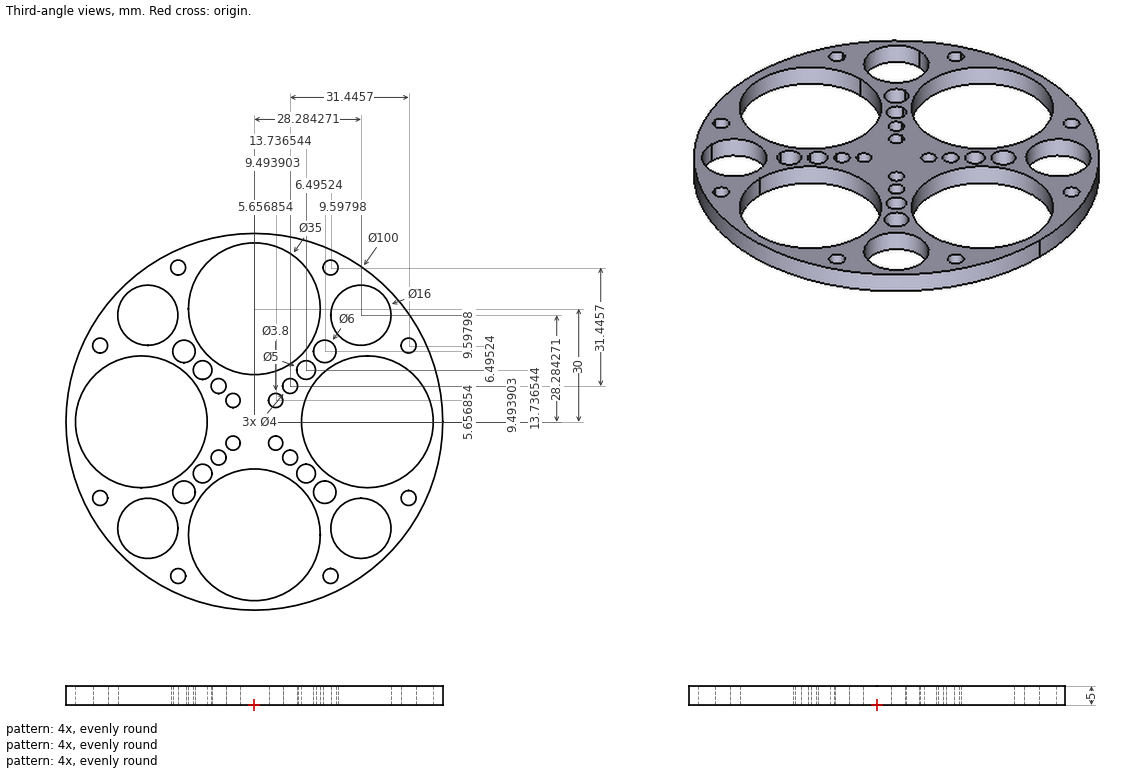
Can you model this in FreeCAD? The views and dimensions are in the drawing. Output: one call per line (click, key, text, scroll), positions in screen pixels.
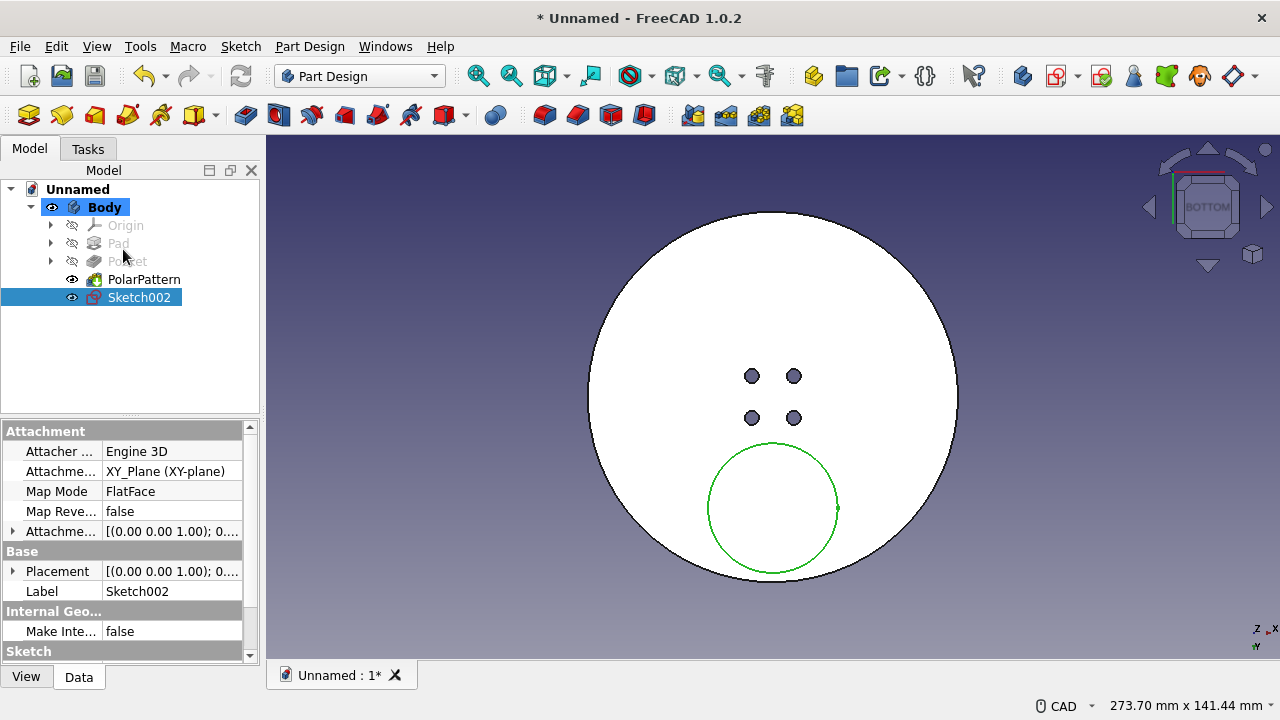
click(246, 116)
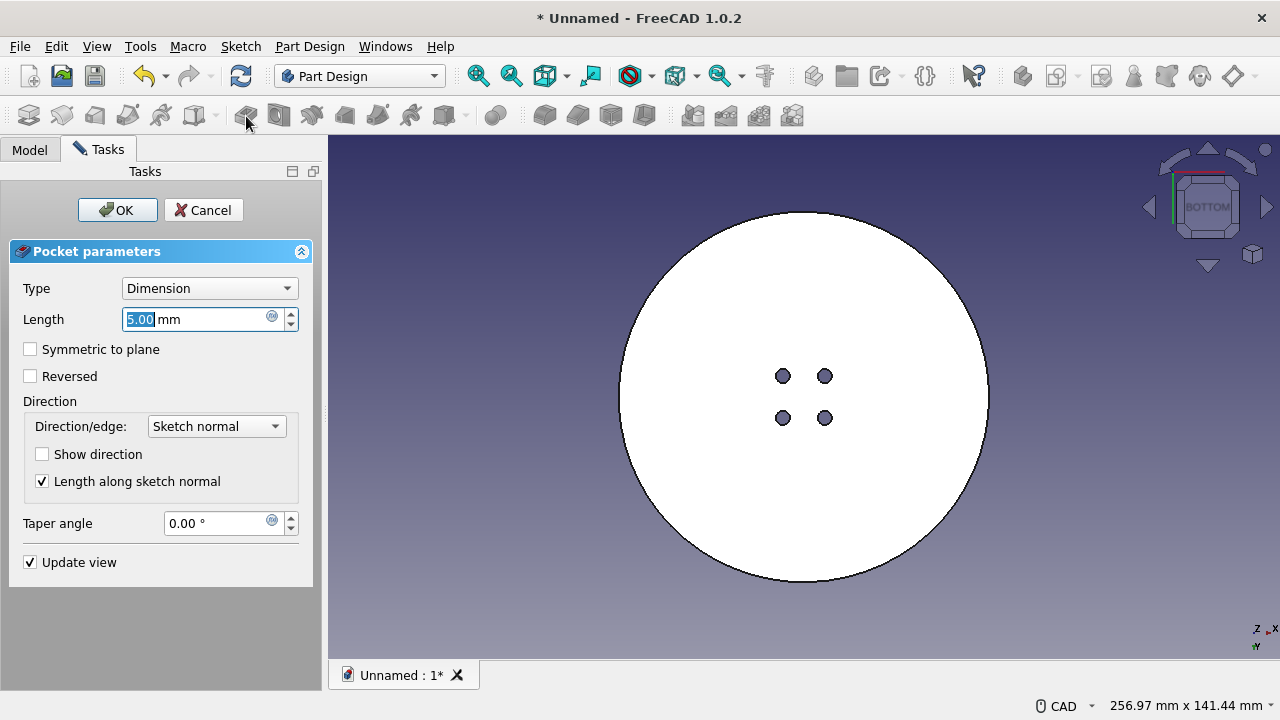
click(210, 288)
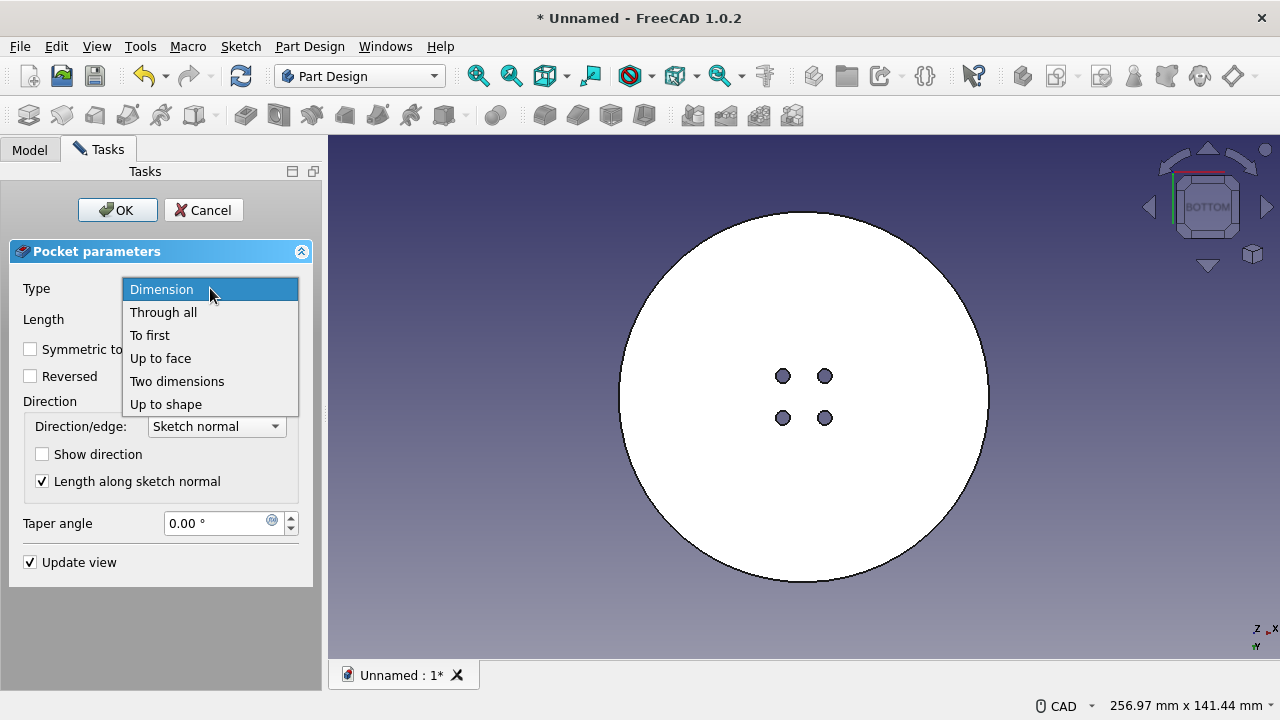
click(208, 312)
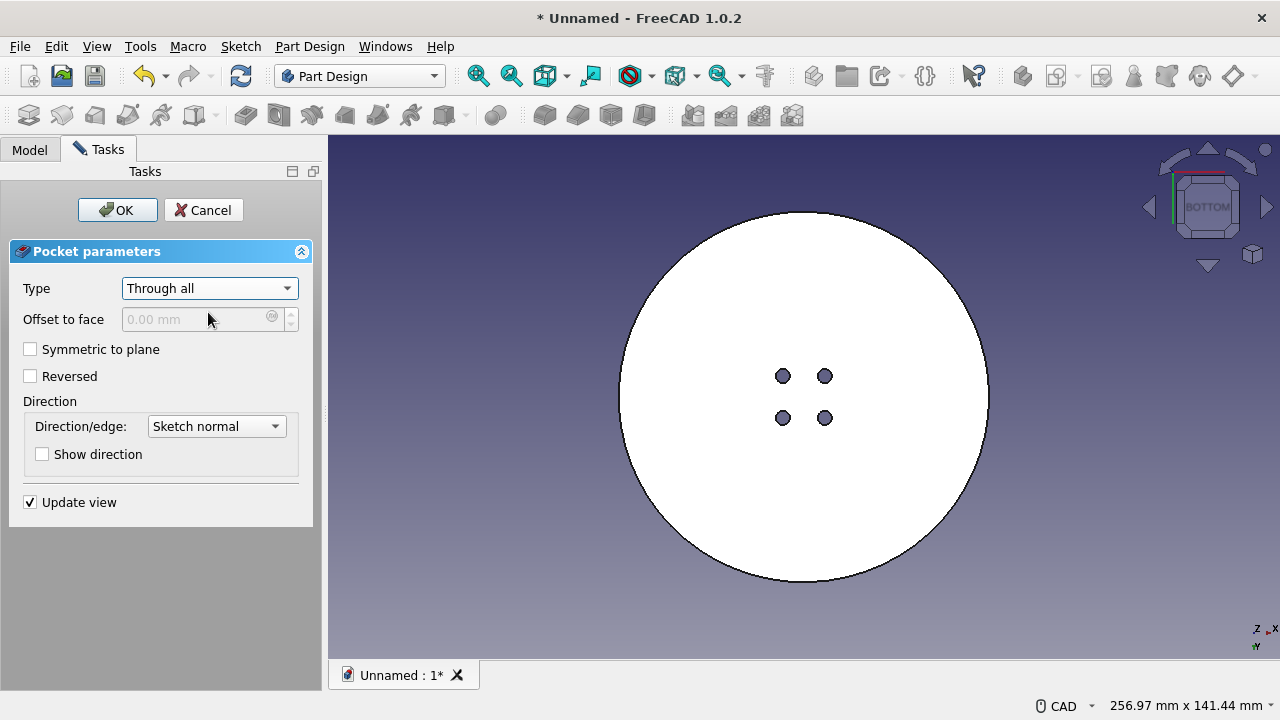
click(31, 376)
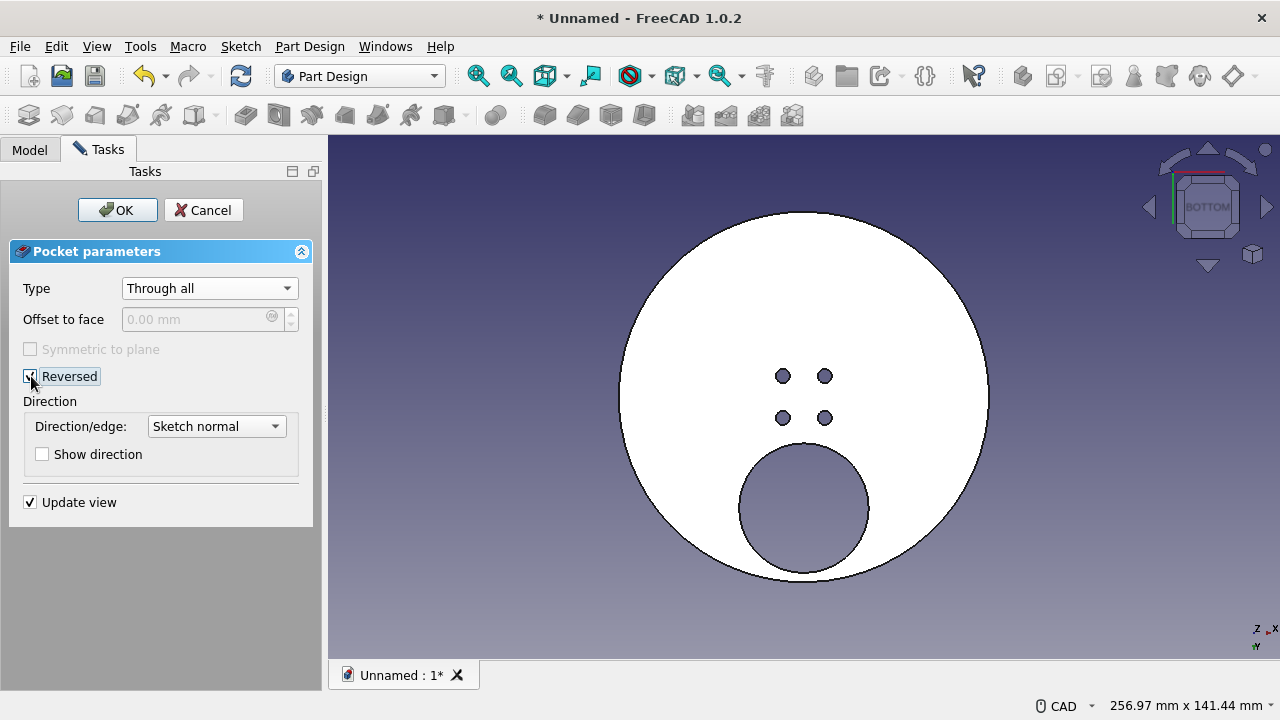
click(118, 210)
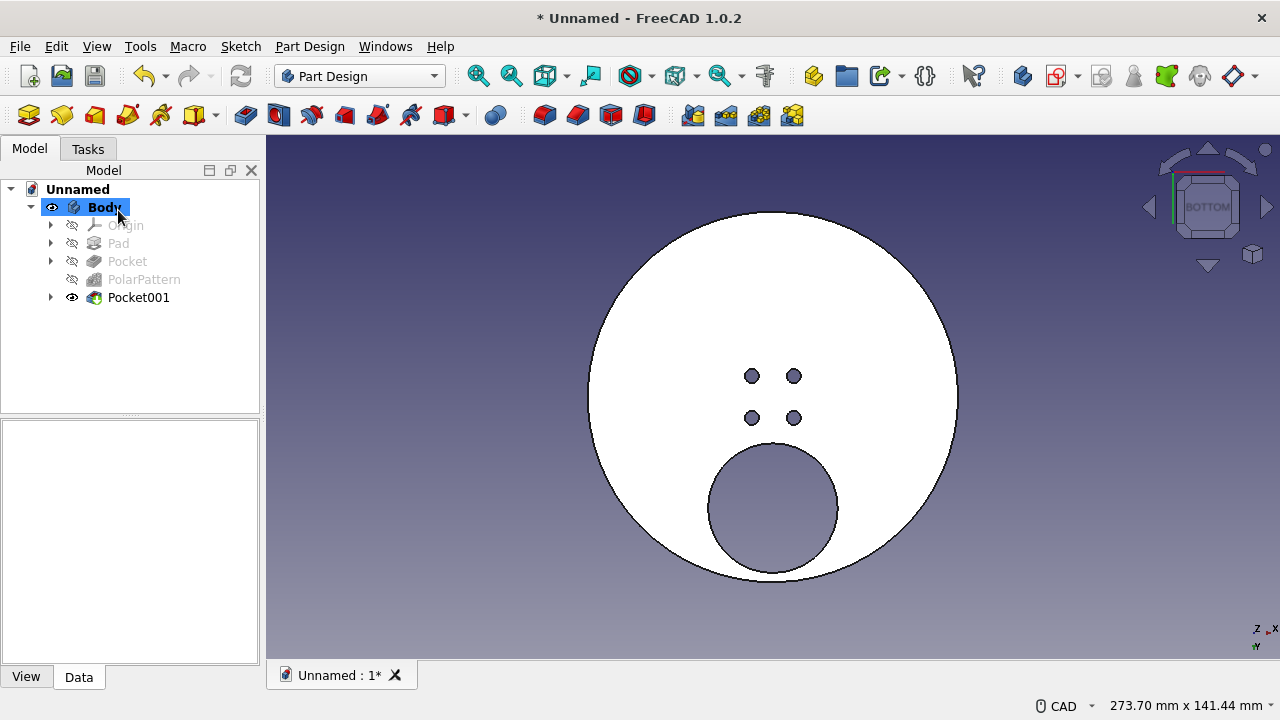
click(117, 297)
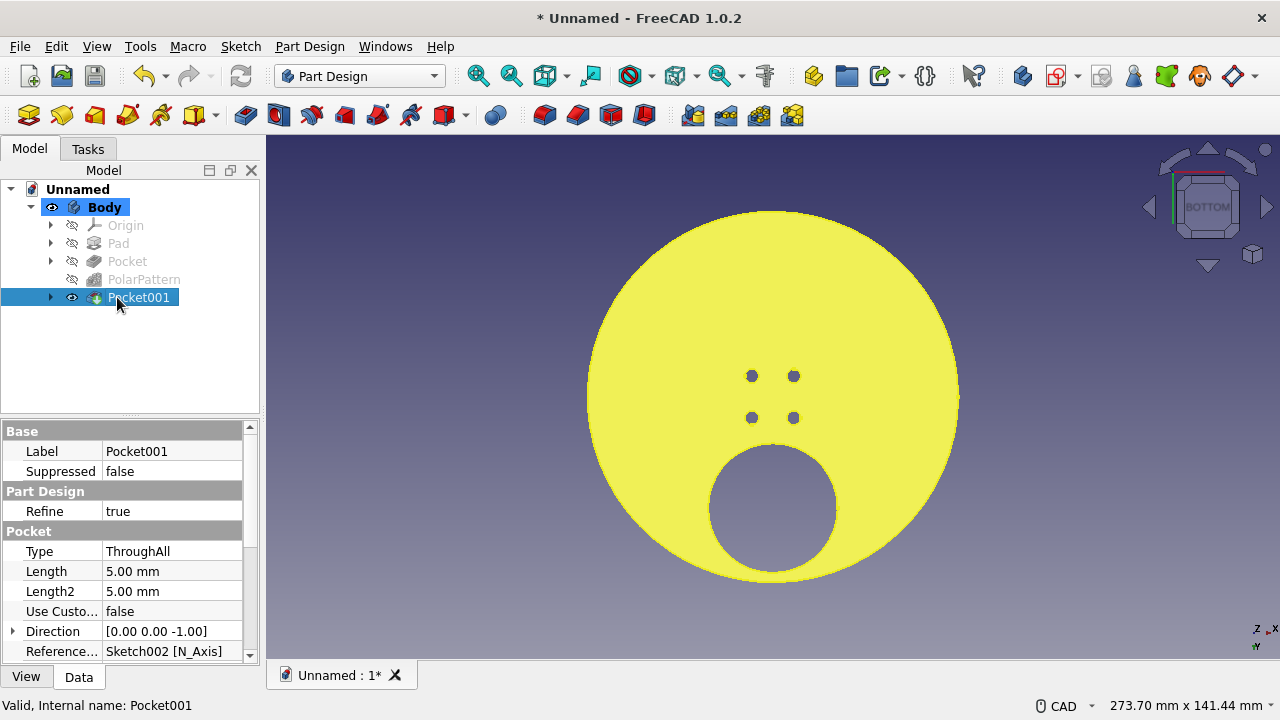
click(759, 116)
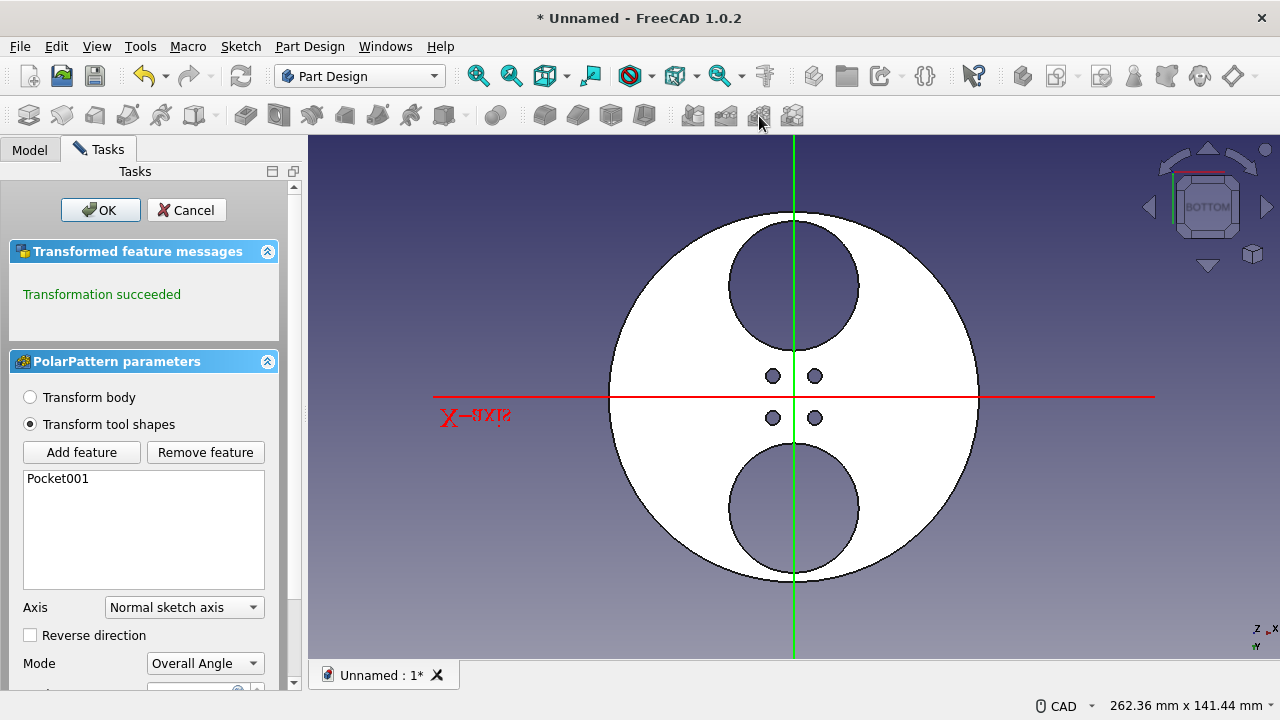
click(185, 608)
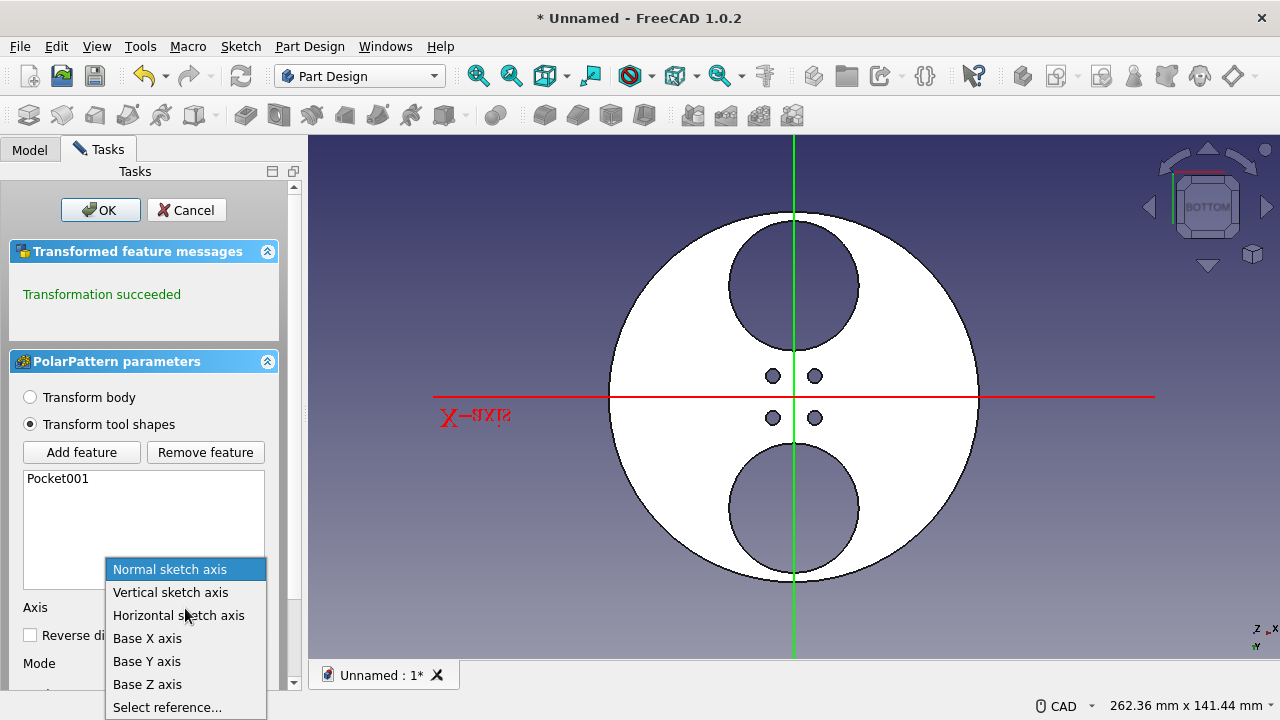
click(184, 684)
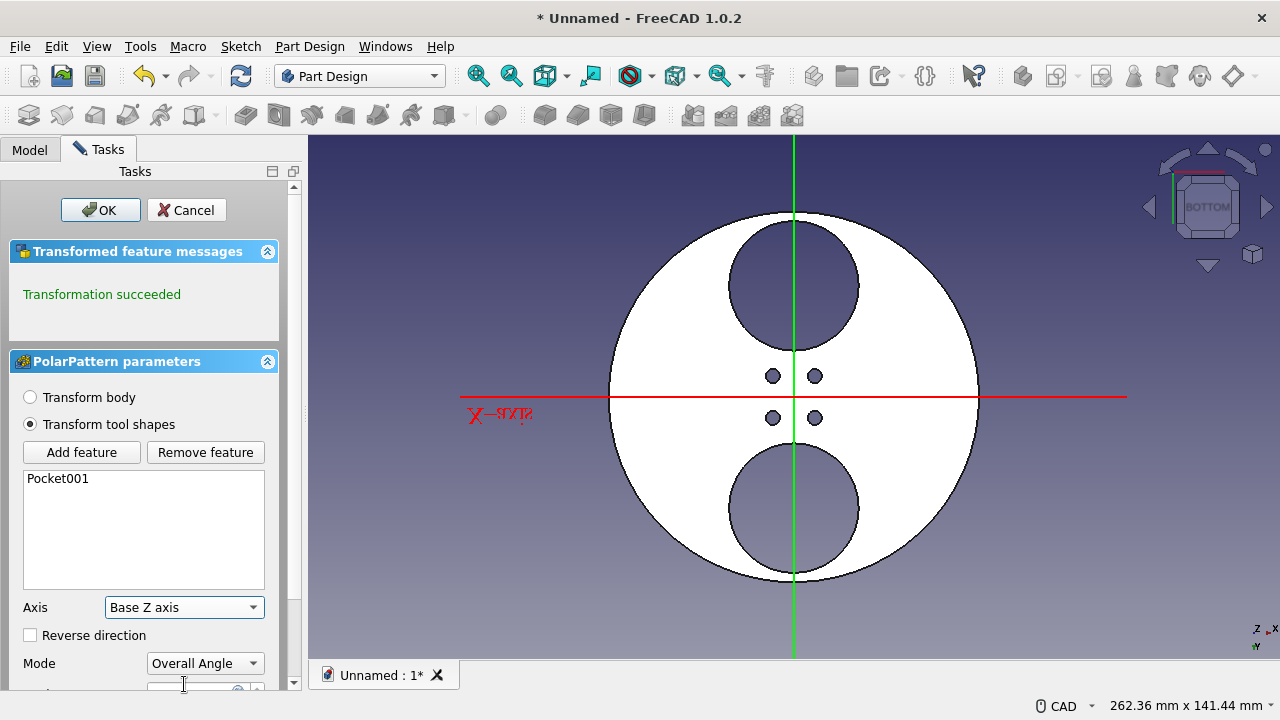
scroll(294, 436, down, 2)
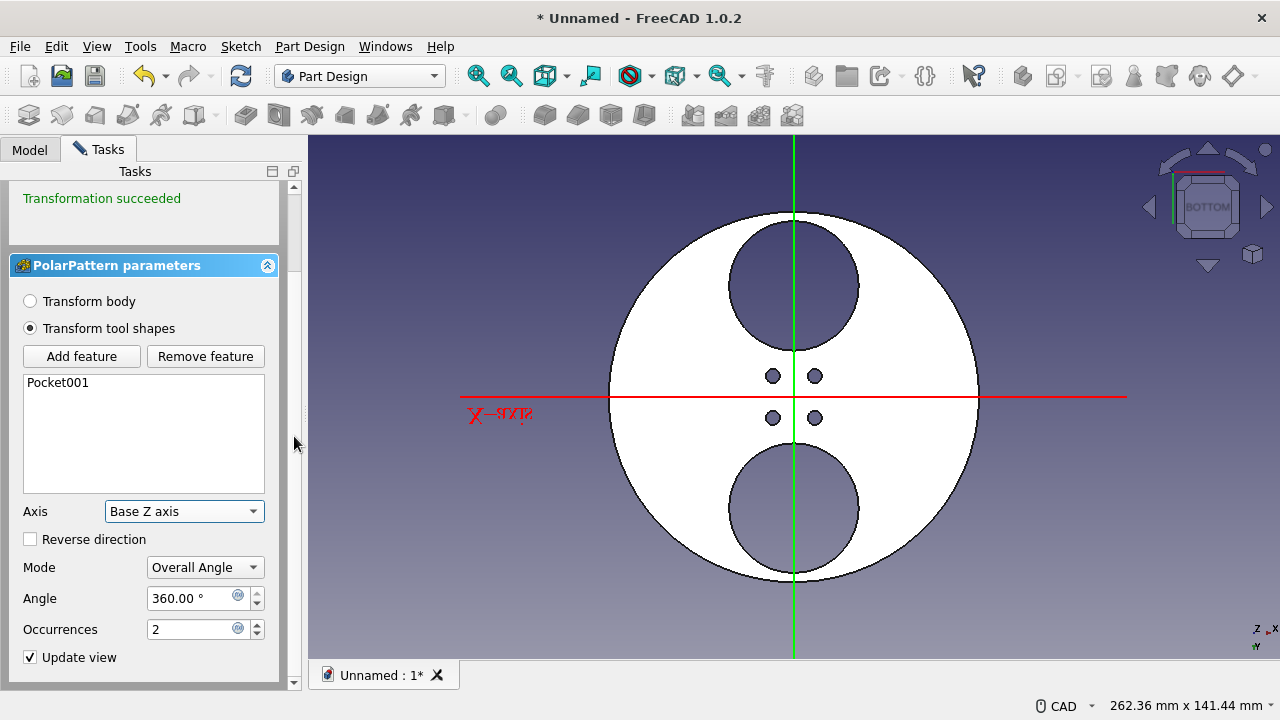
triple_click(199, 630)